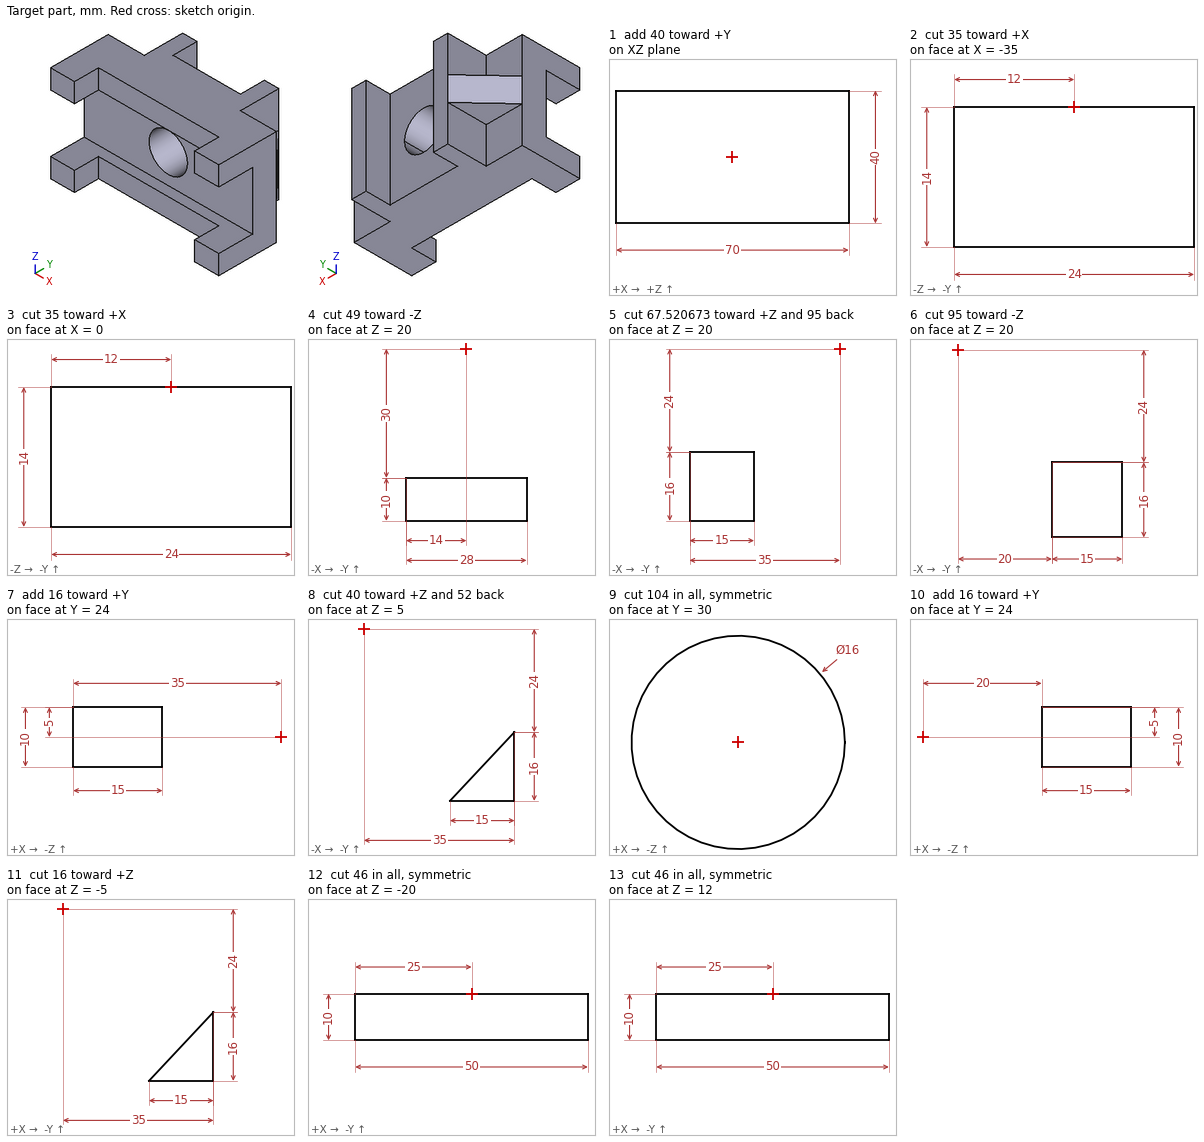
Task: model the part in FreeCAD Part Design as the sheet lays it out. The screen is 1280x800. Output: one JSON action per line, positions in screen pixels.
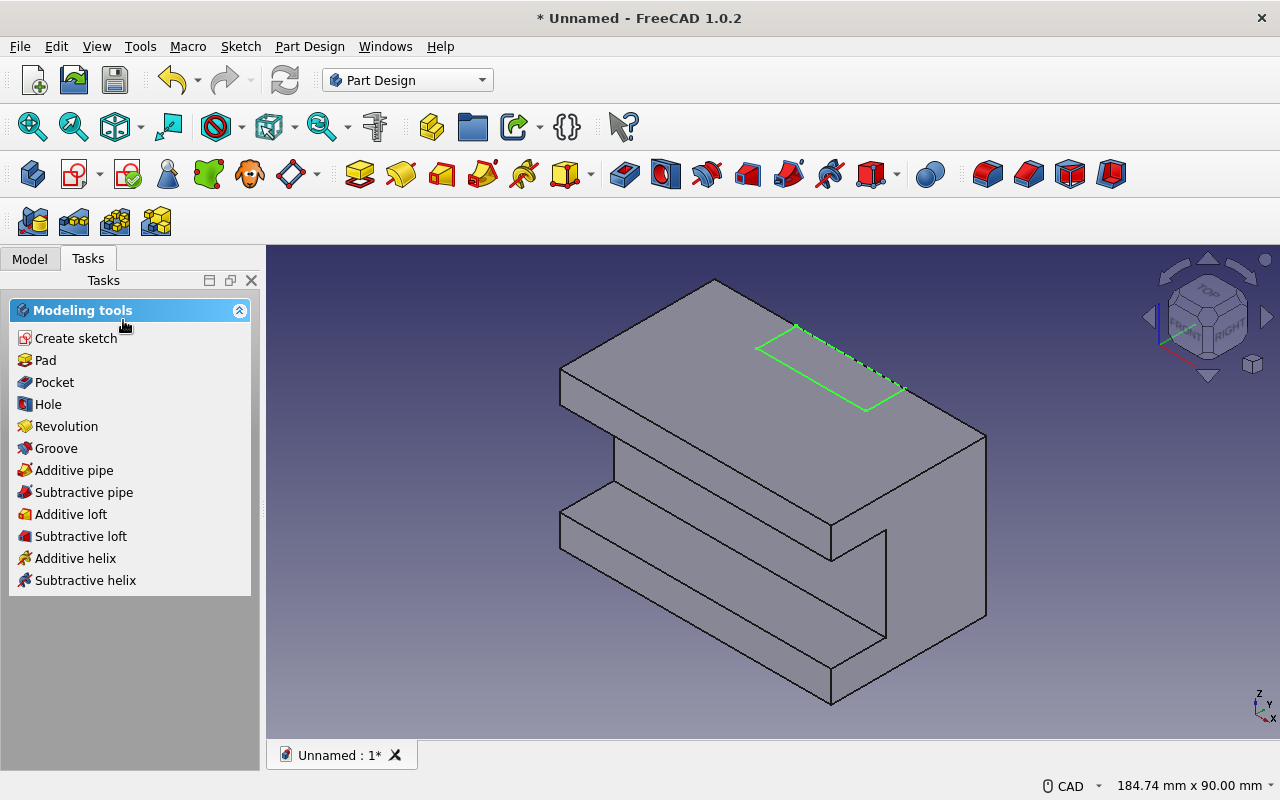
{"action": "left_click", "coordinate": [625, 174]}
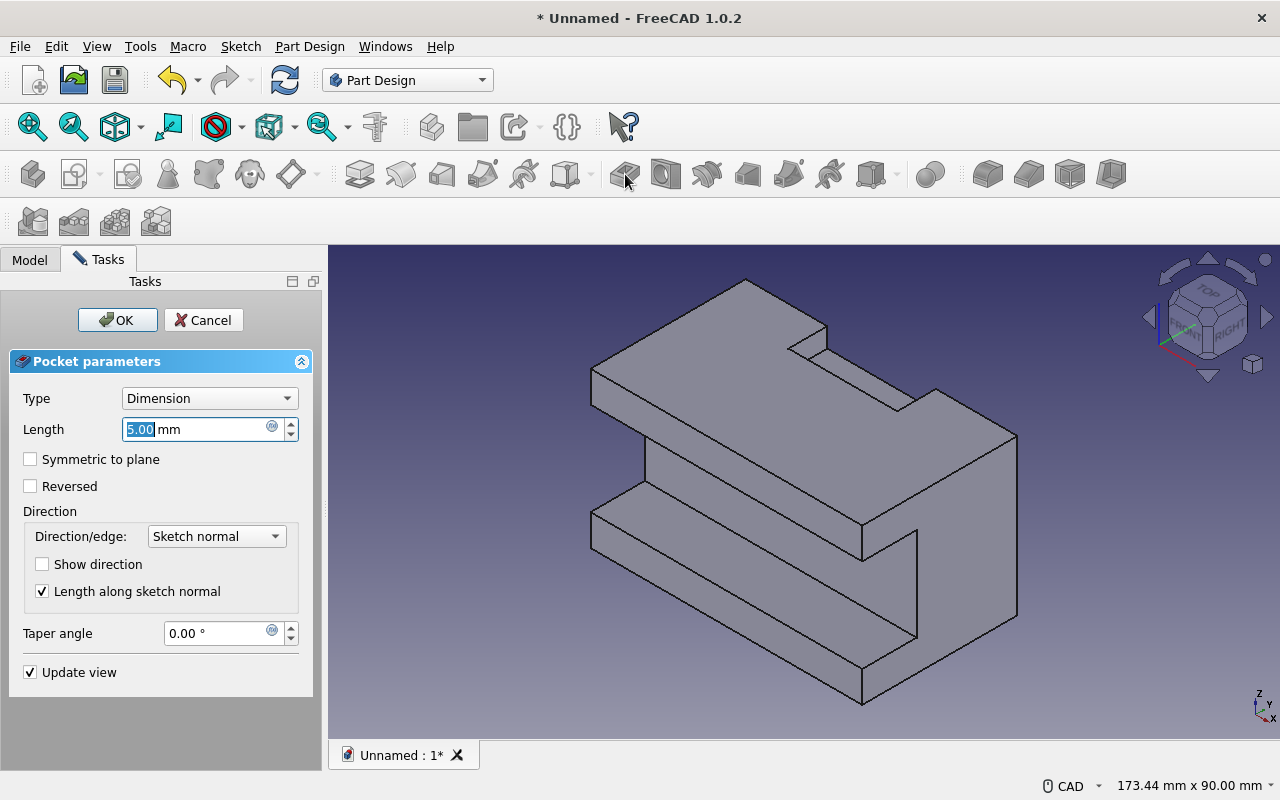
{"action": "type", "text": "49"}
{"action": "key", "text": "Tab"}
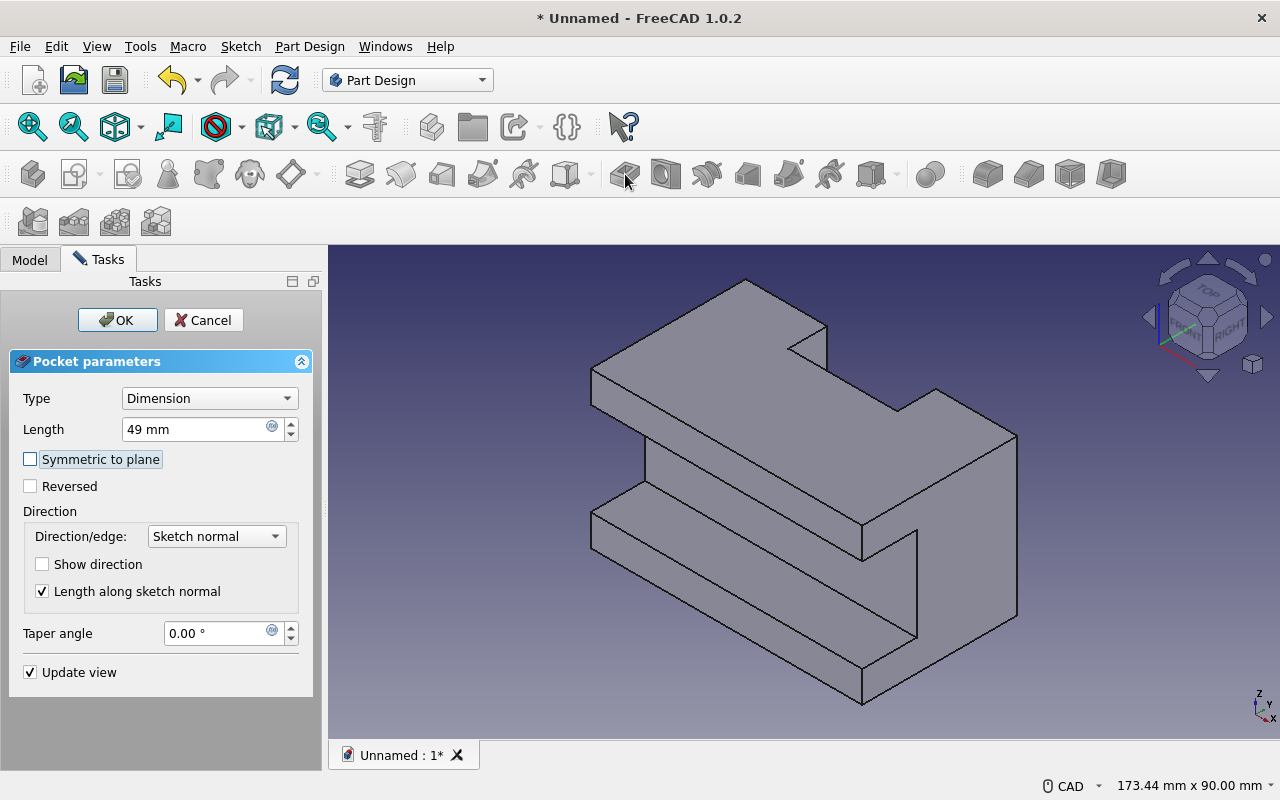
{"action": "left_click", "coordinate": [118, 320]}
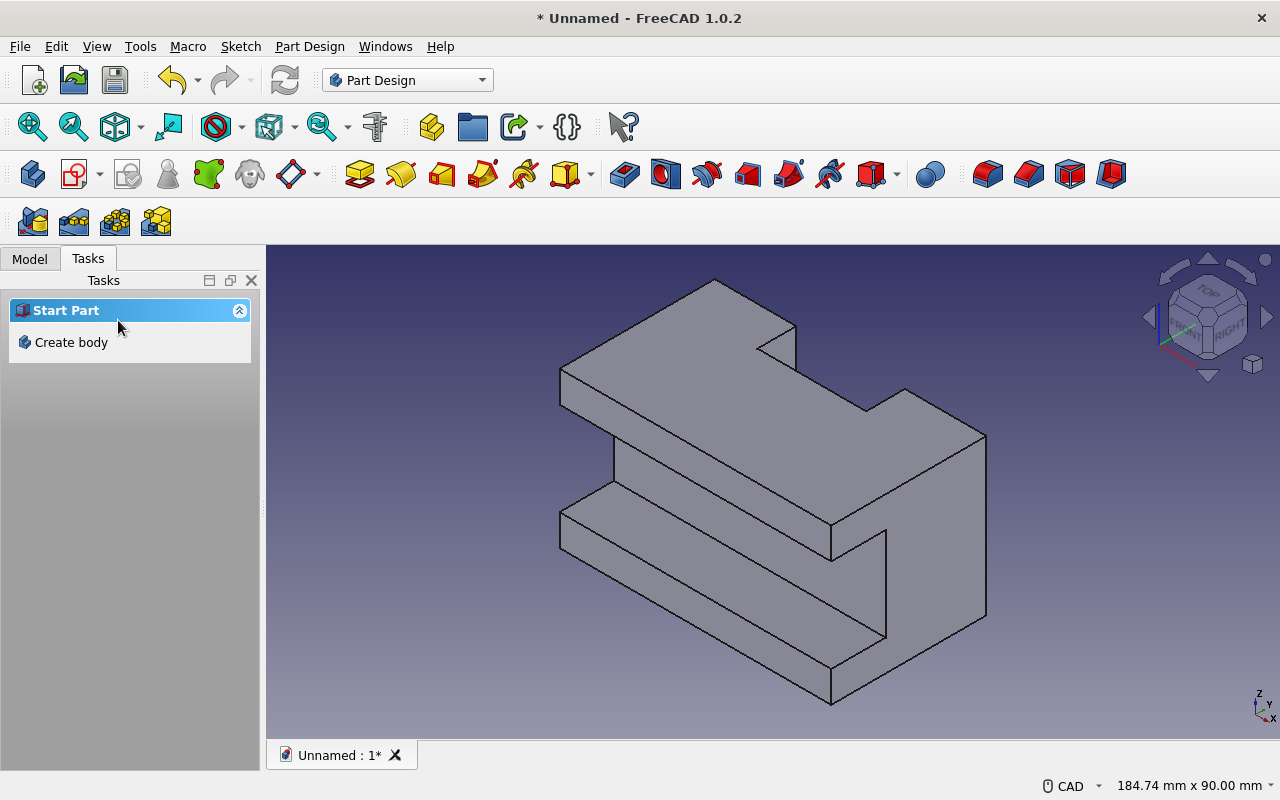
{"action": "left_click", "coordinate": [828, 459]}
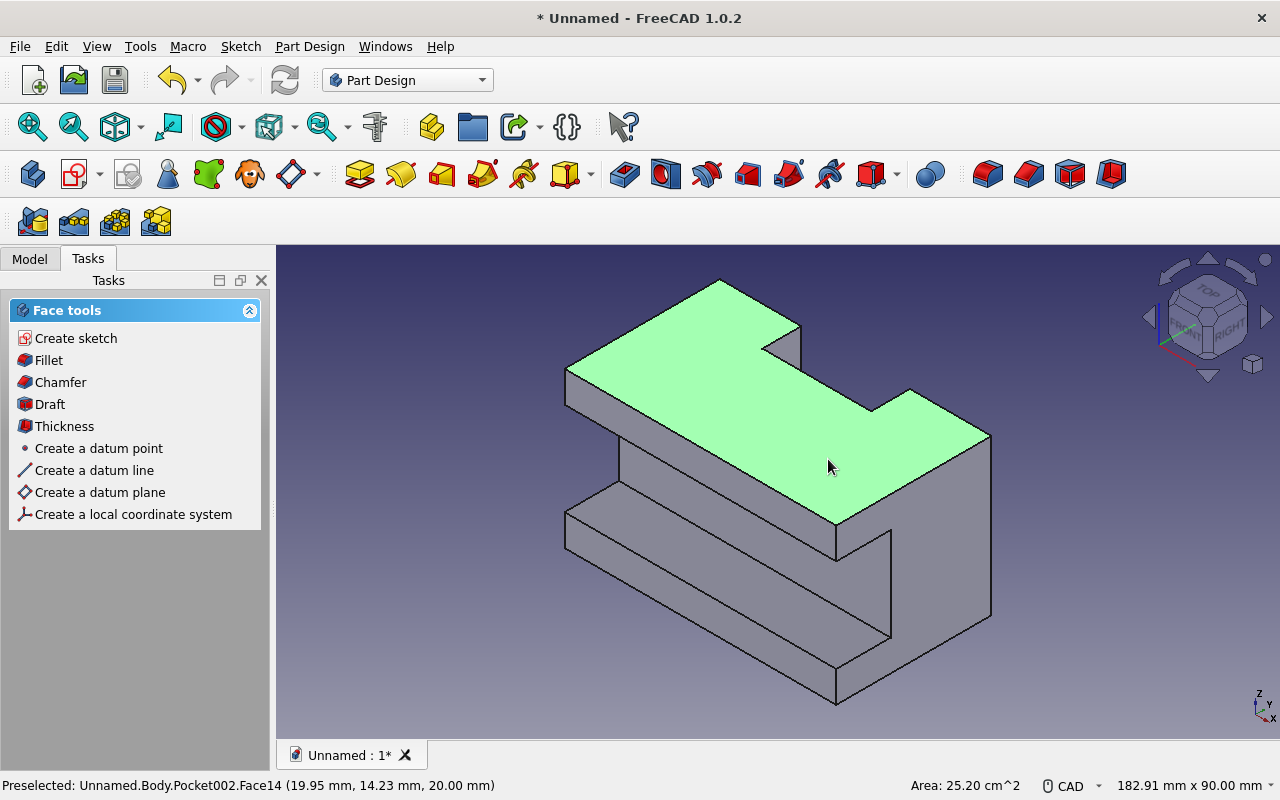
{"action": "left_click", "coordinate": [74, 174]}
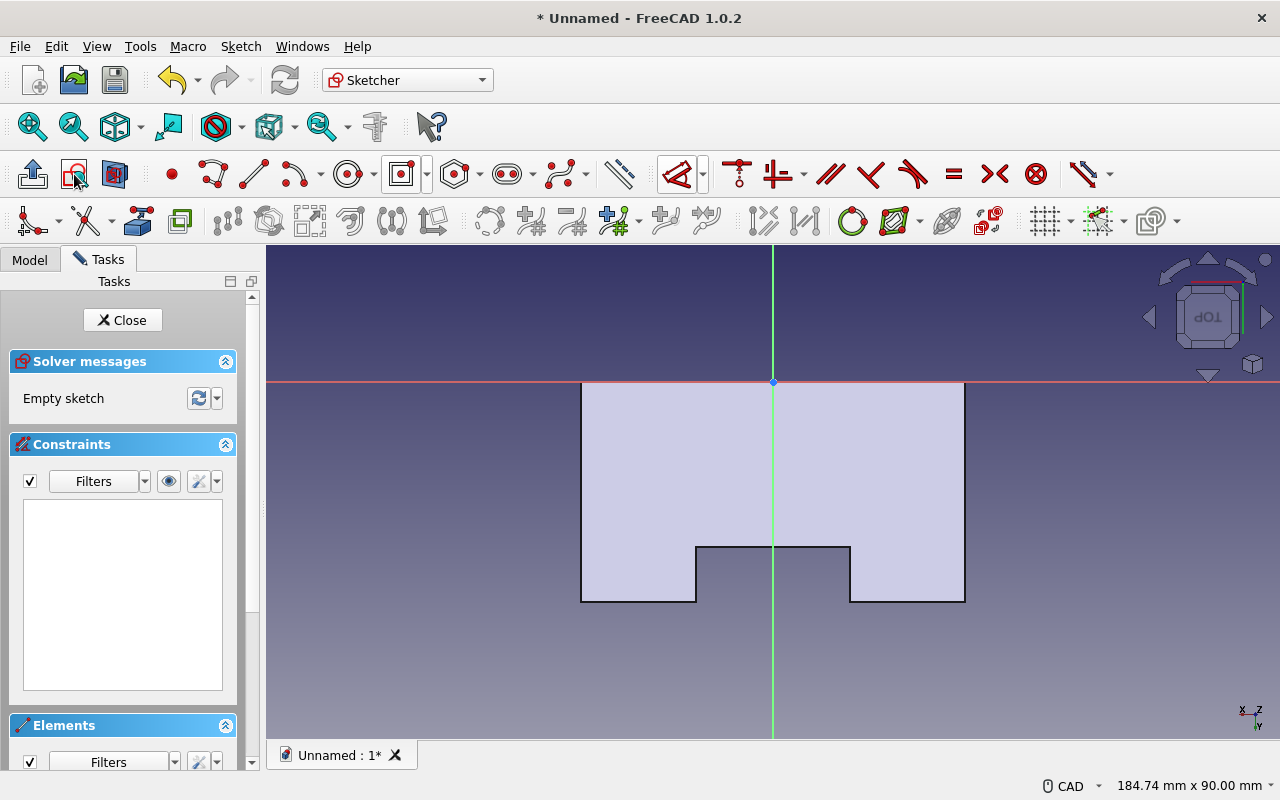
{"action": "scroll", "coordinate": [587, 586], "scroll_direction": "up", "scroll_amount": 6}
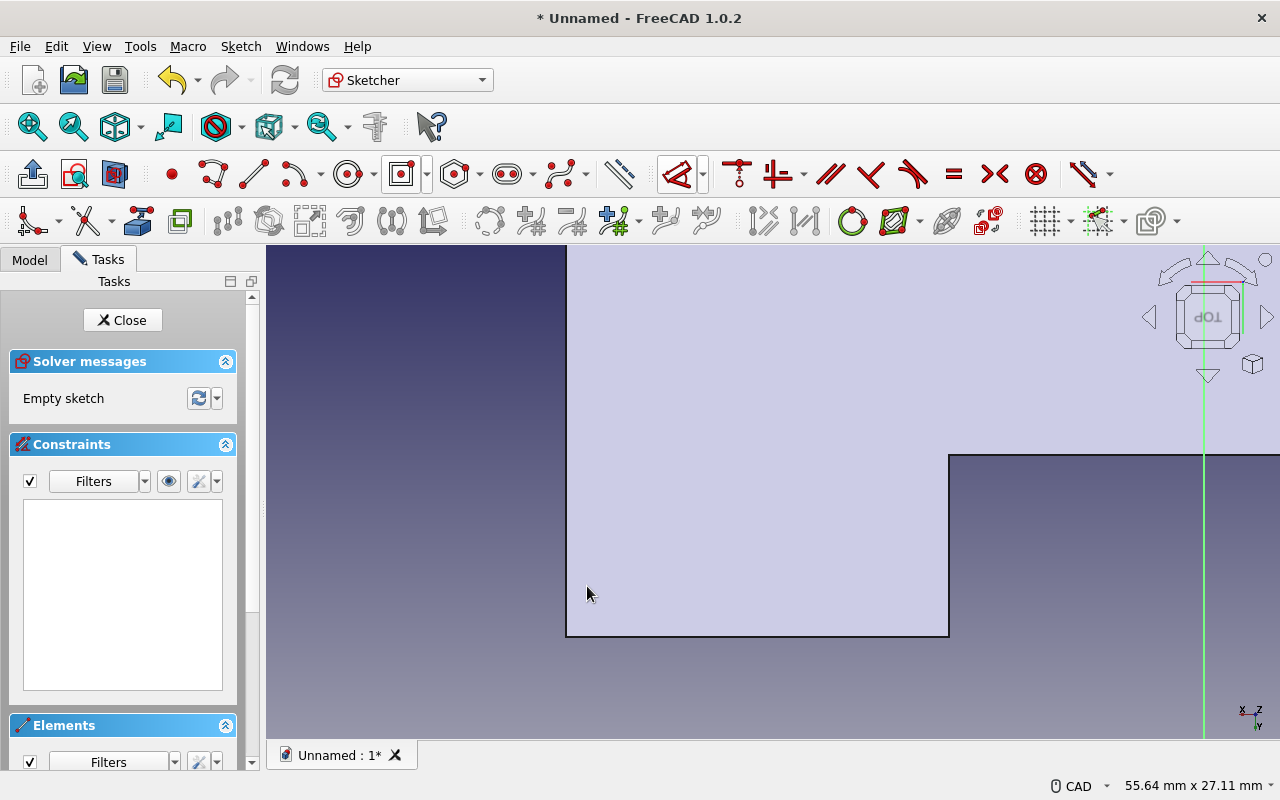
{"action": "key", "text": "g r"}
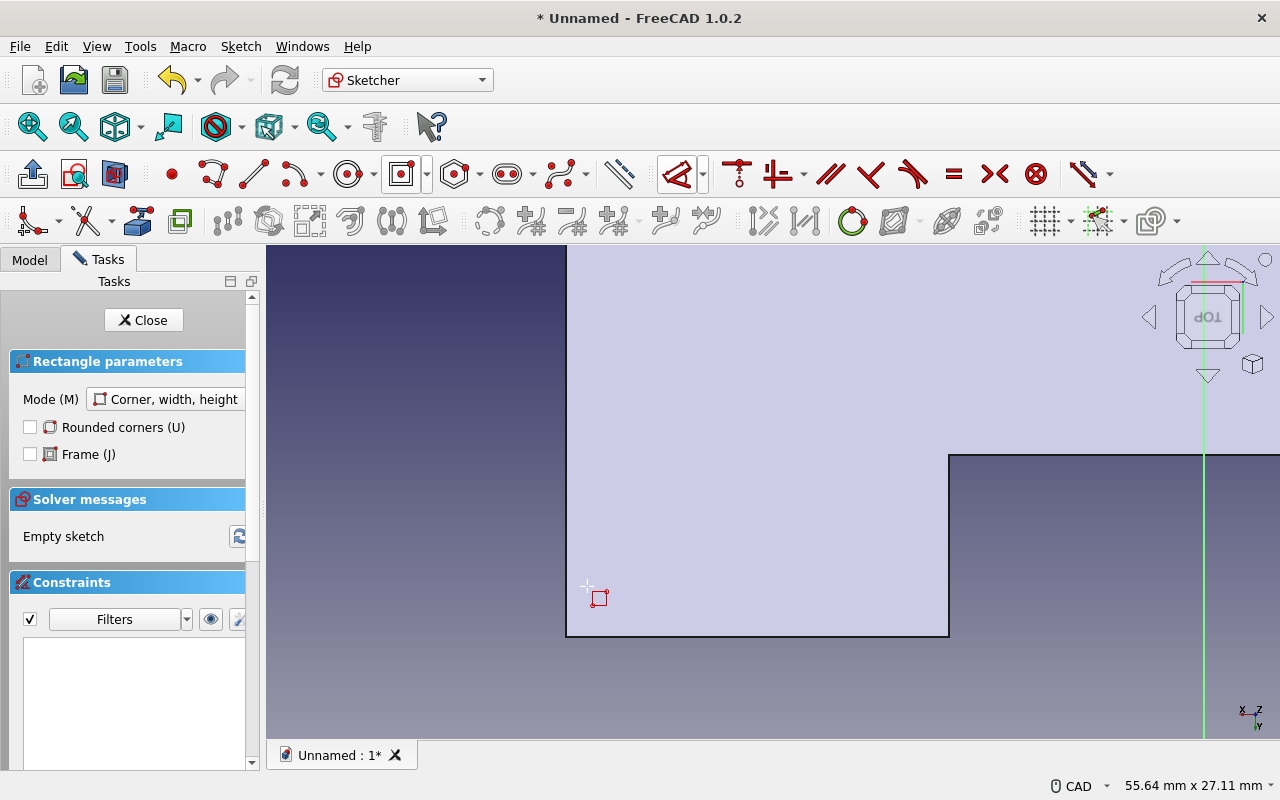
{"action": "left_click", "coordinate": [566, 345]}
{"action": "left_click", "coordinate": [839, 637]}
{"action": "key", "text": "Escape"}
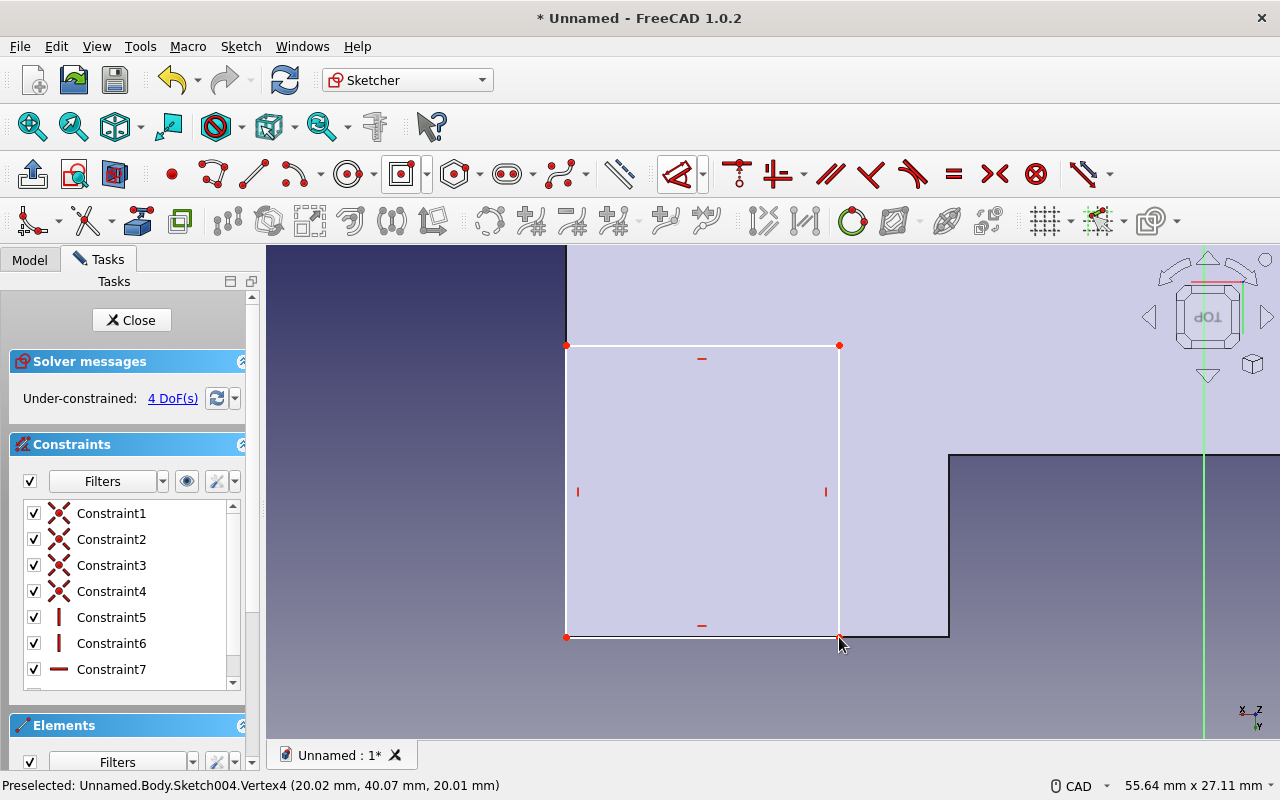
{"action": "left_click", "coordinate": [566, 434]}